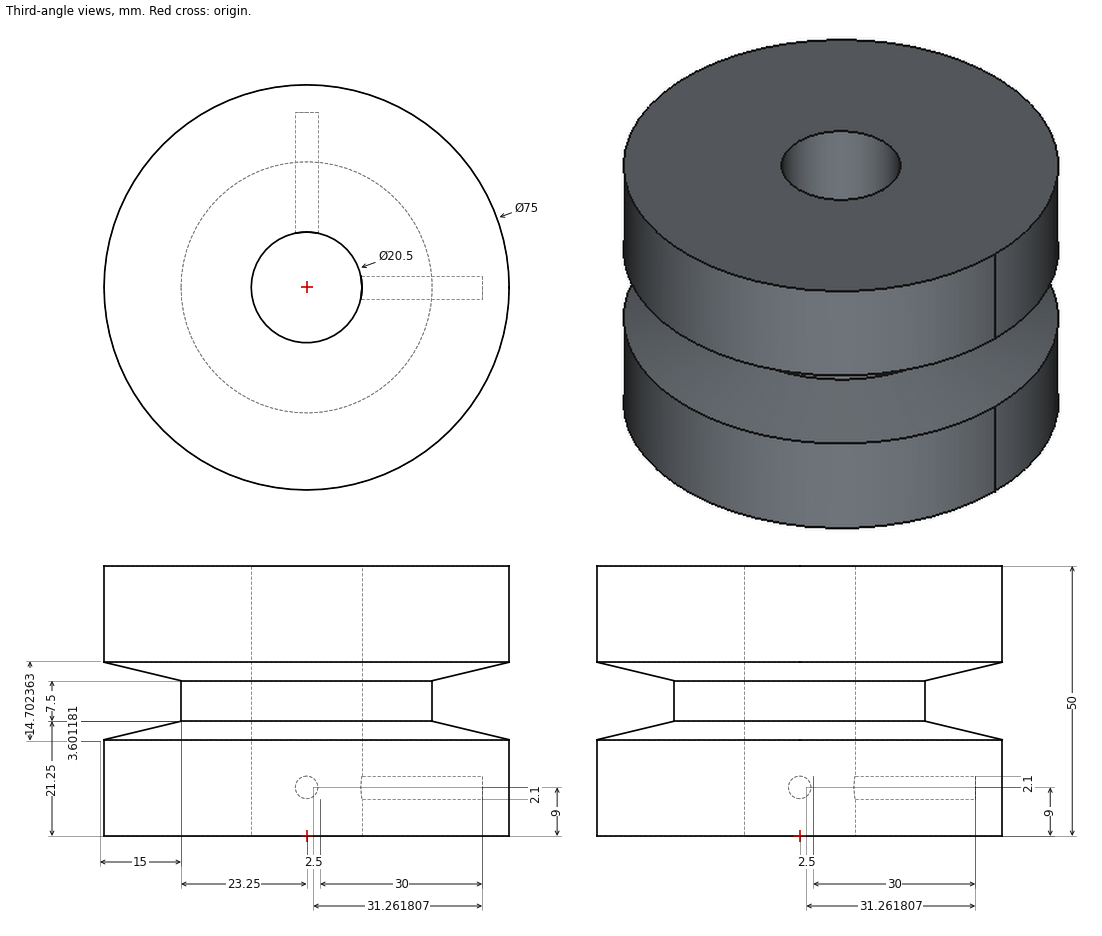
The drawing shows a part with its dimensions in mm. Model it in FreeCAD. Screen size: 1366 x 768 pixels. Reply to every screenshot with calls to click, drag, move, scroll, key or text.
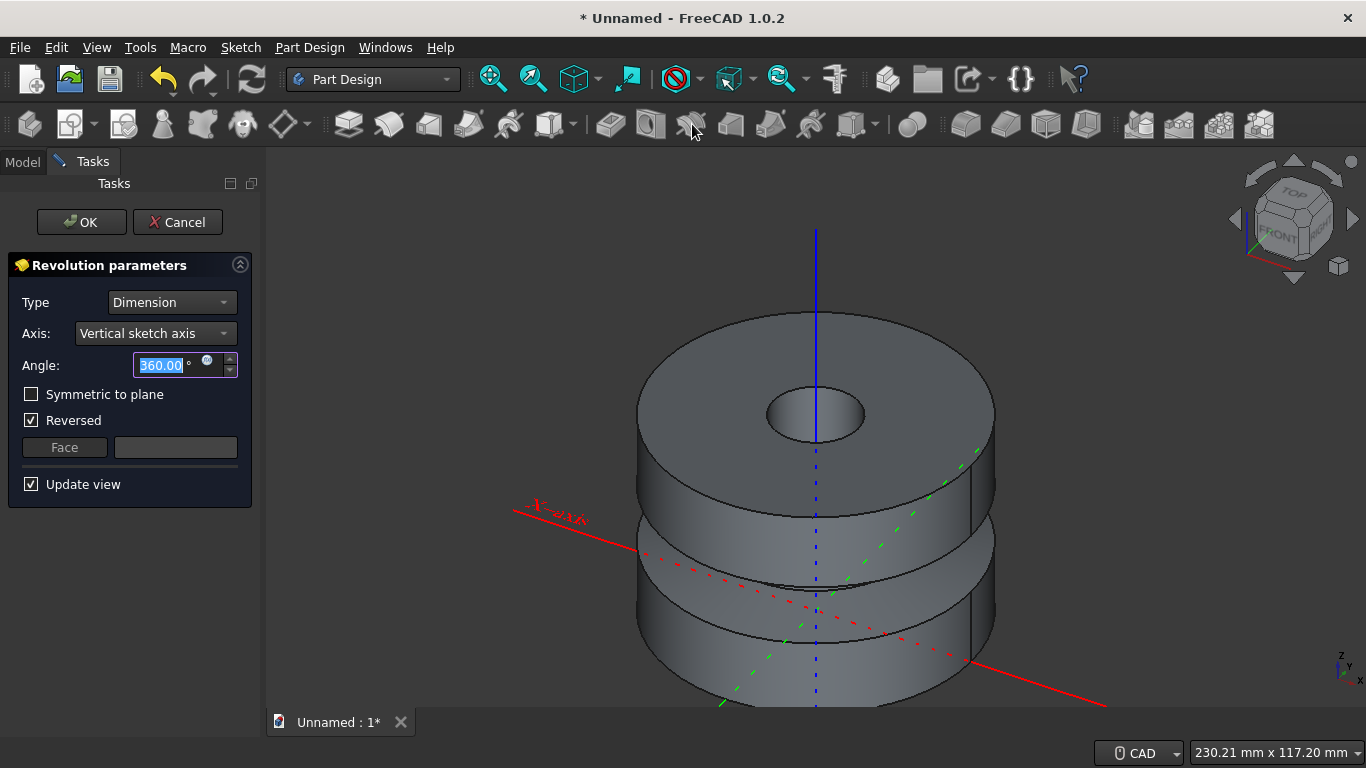
click(82, 222)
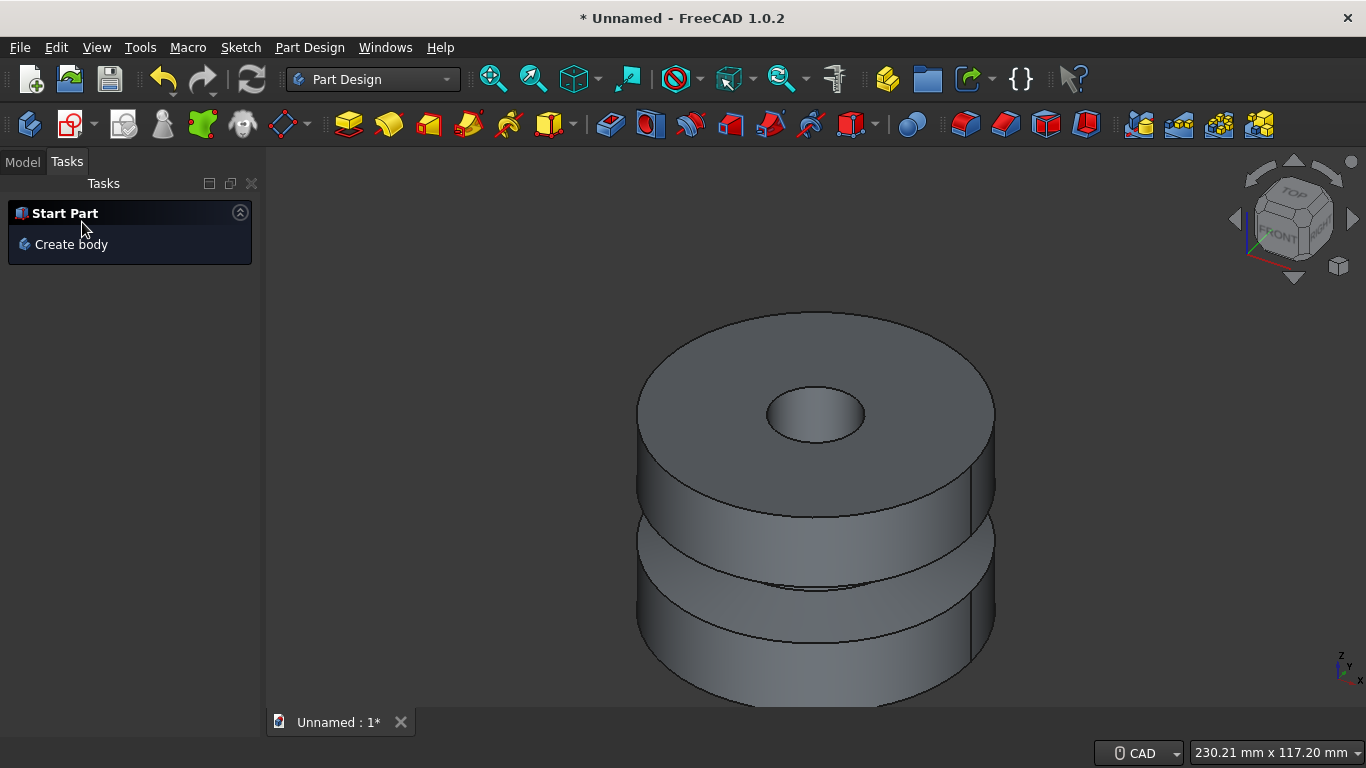
click(494, 80)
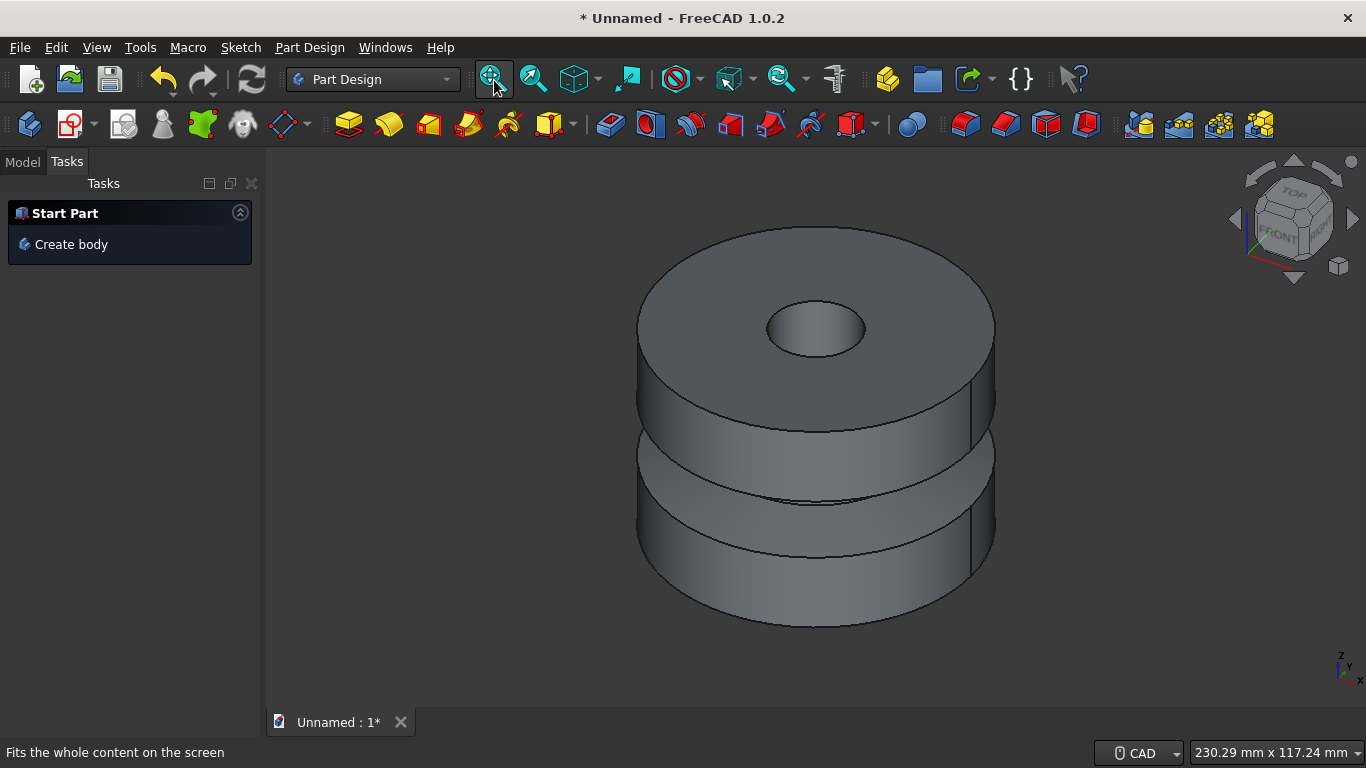
click(70, 124)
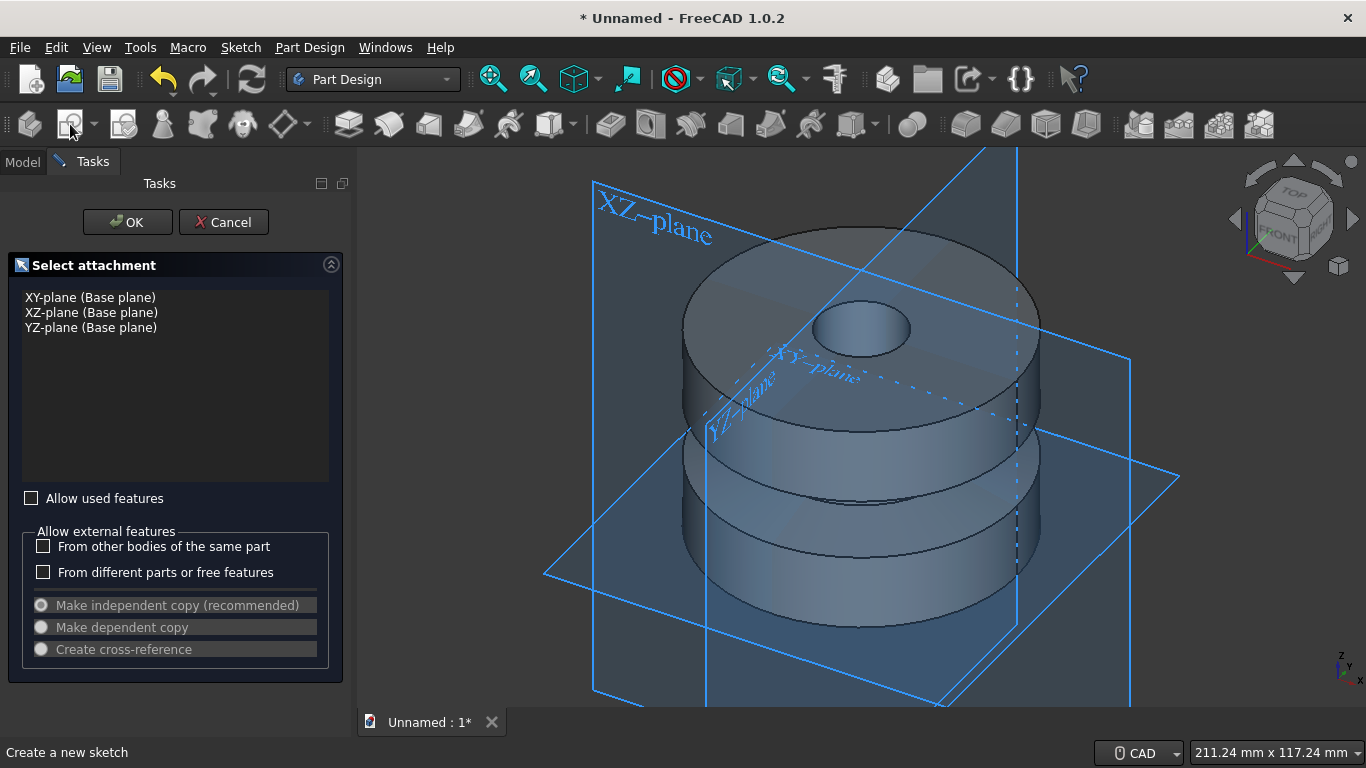
click(82, 328)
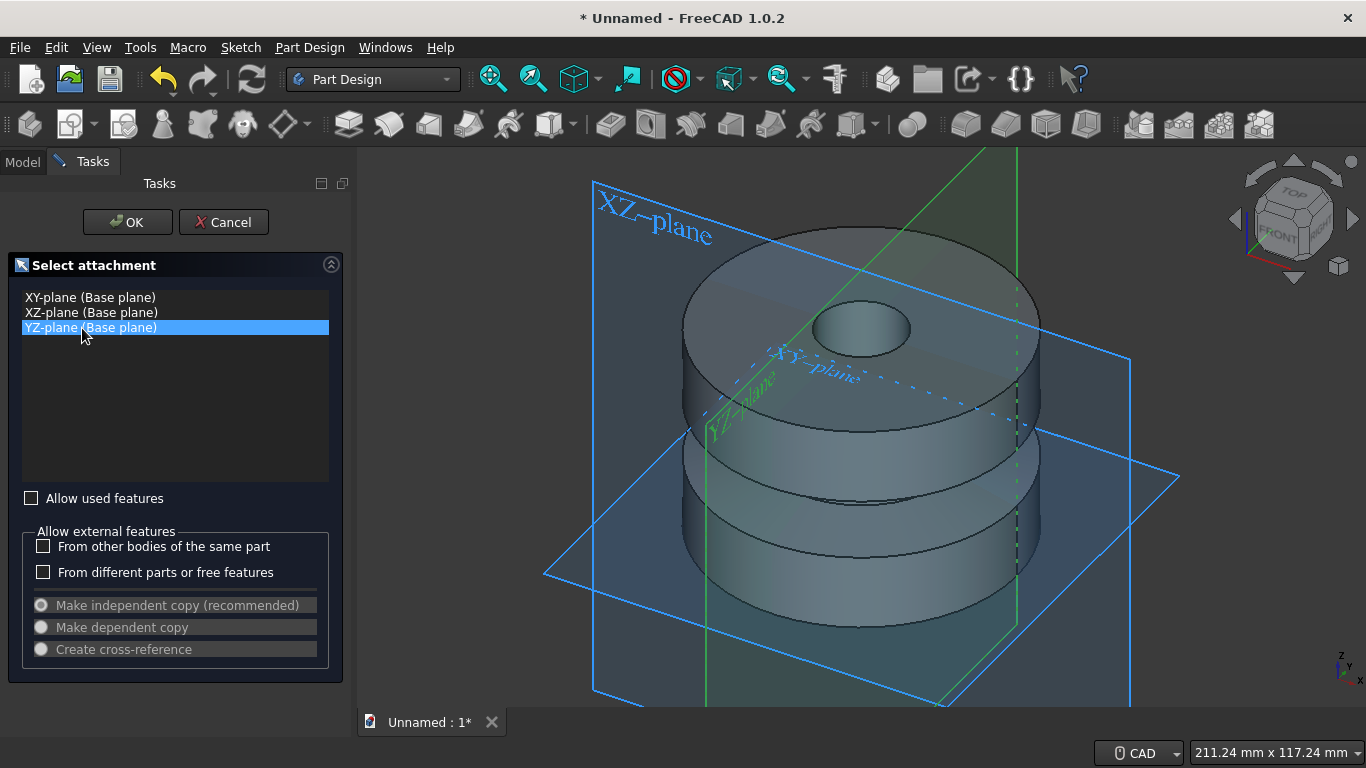
click(128, 222)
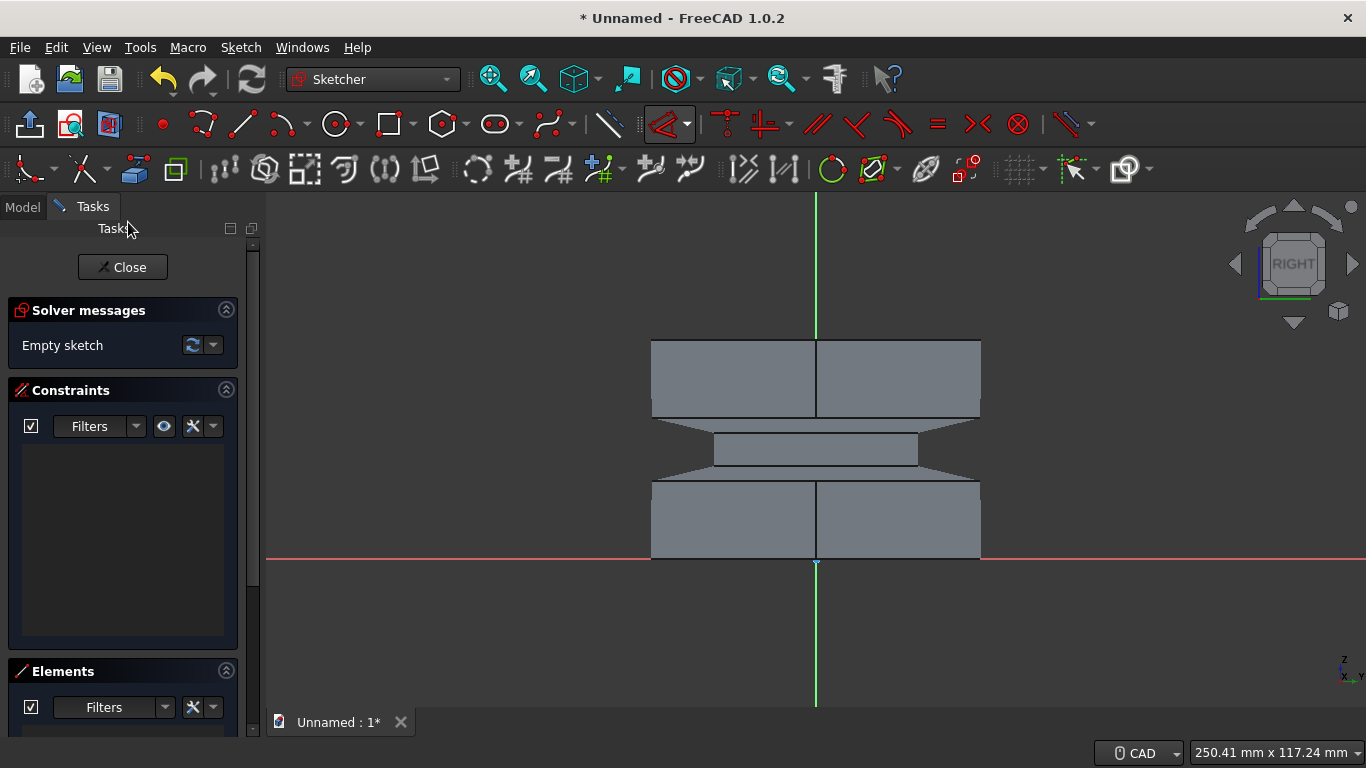
click(110, 124)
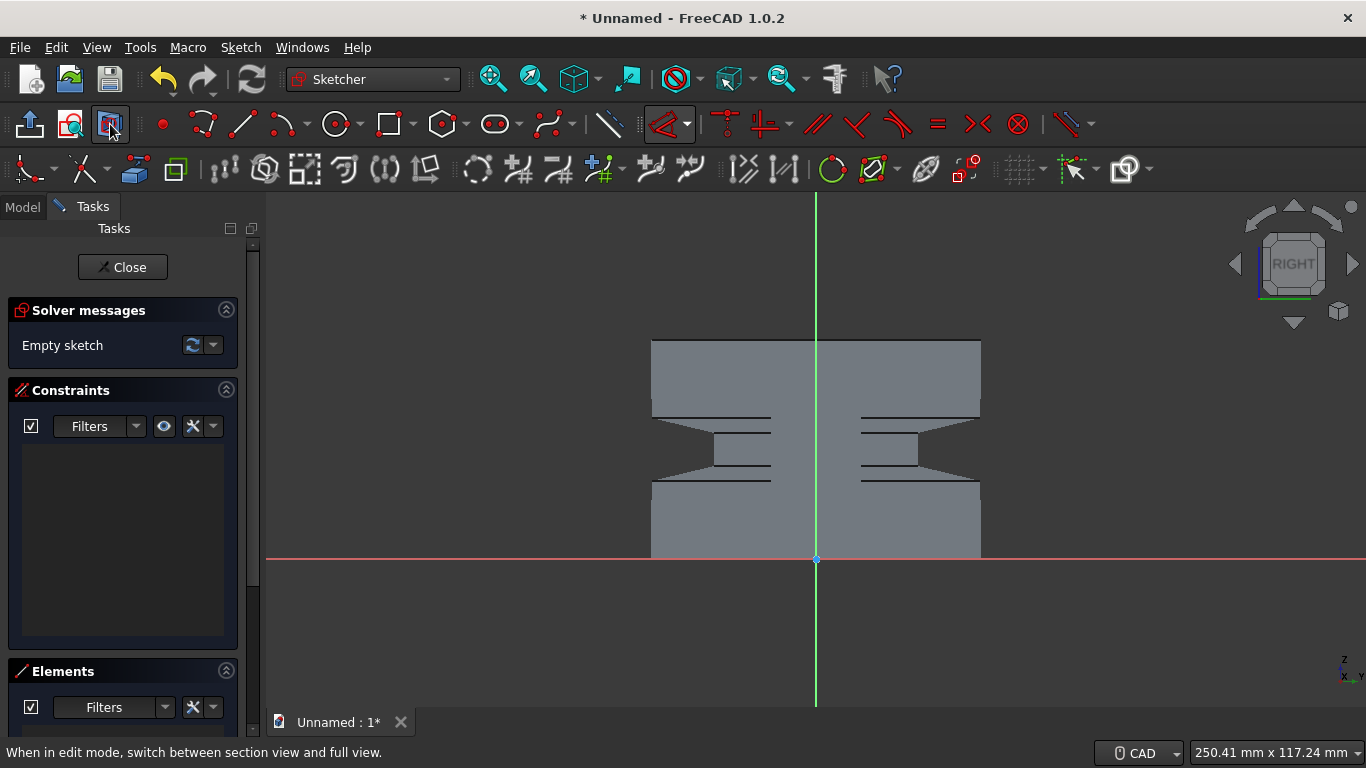
scroll(912, 572, up, 6)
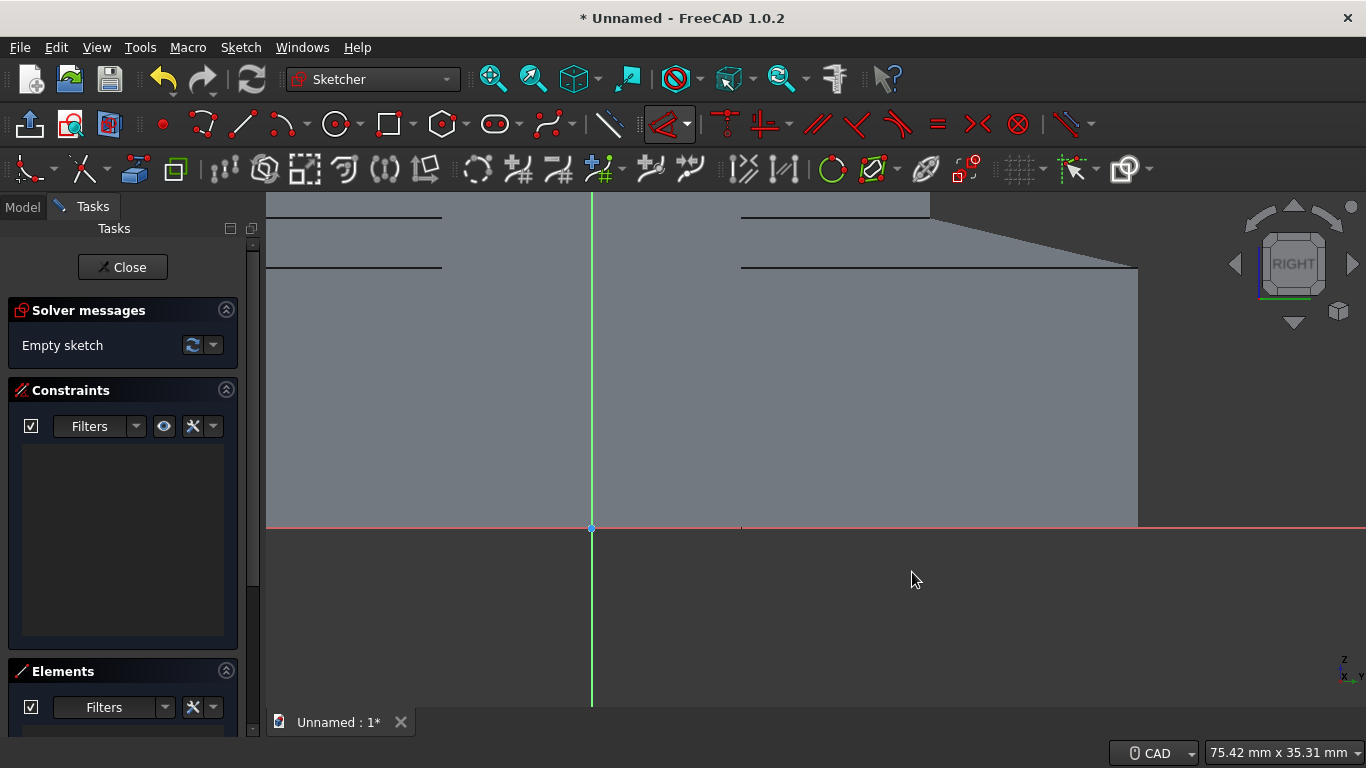
click(204, 124)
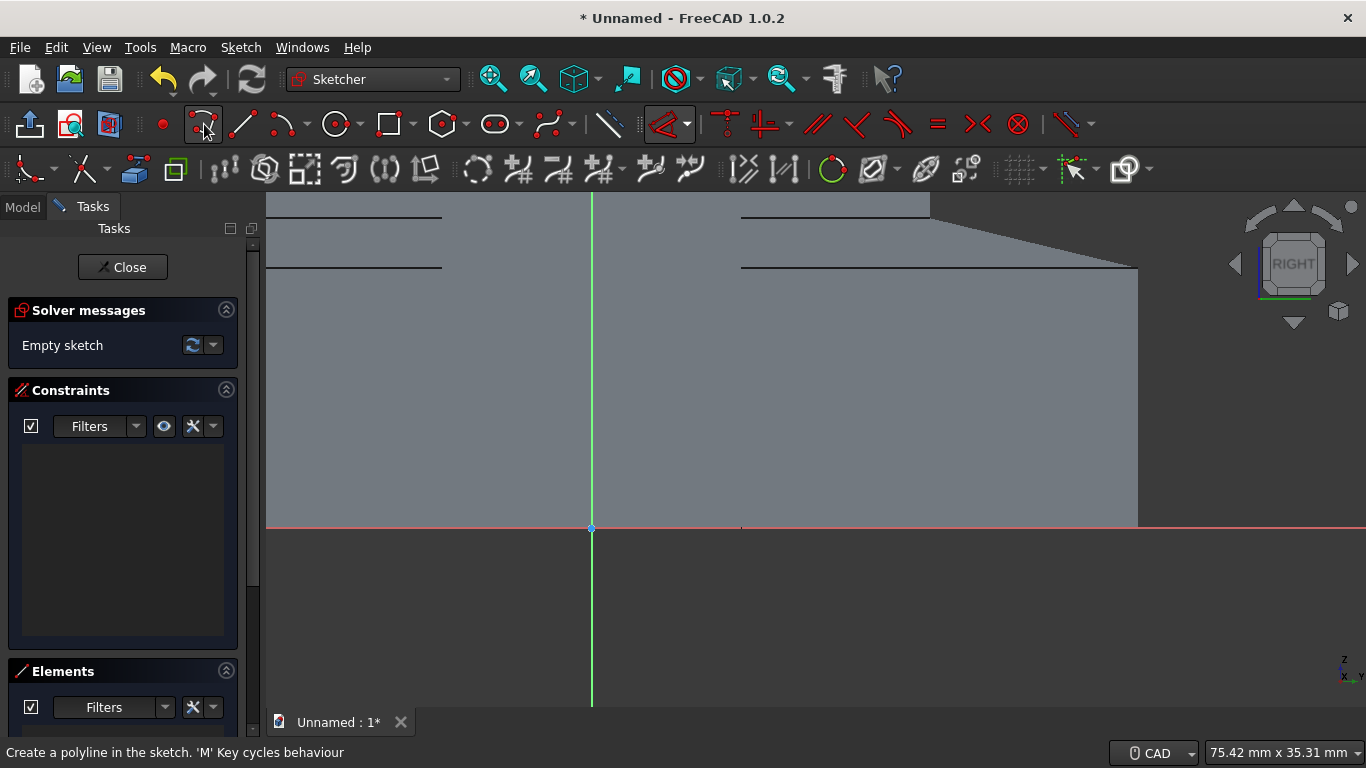
click(610, 397)
click(1066, 397)
click(1066, 366)
click(628, 366)
click(610, 398)